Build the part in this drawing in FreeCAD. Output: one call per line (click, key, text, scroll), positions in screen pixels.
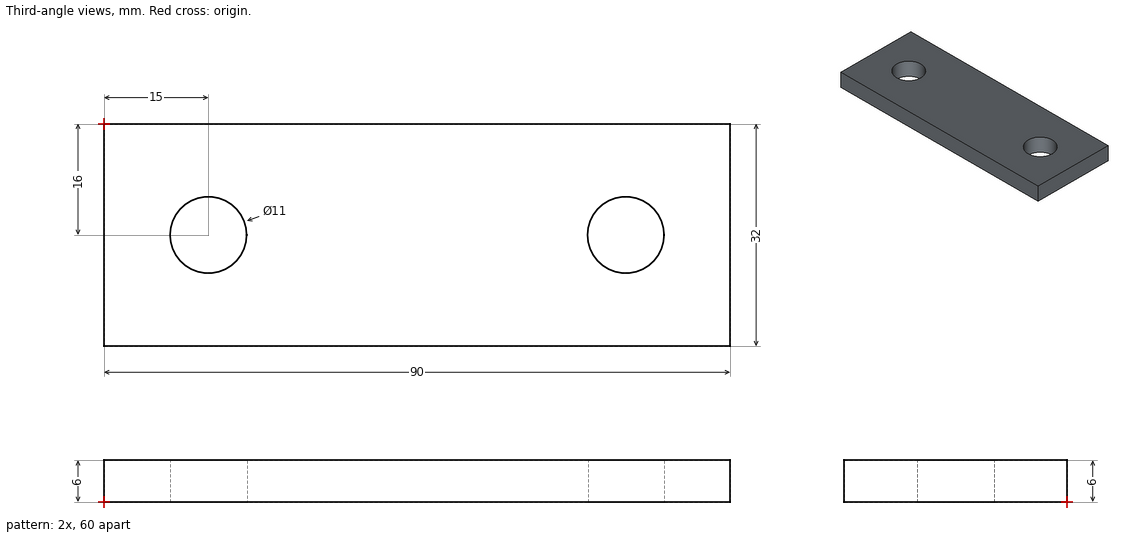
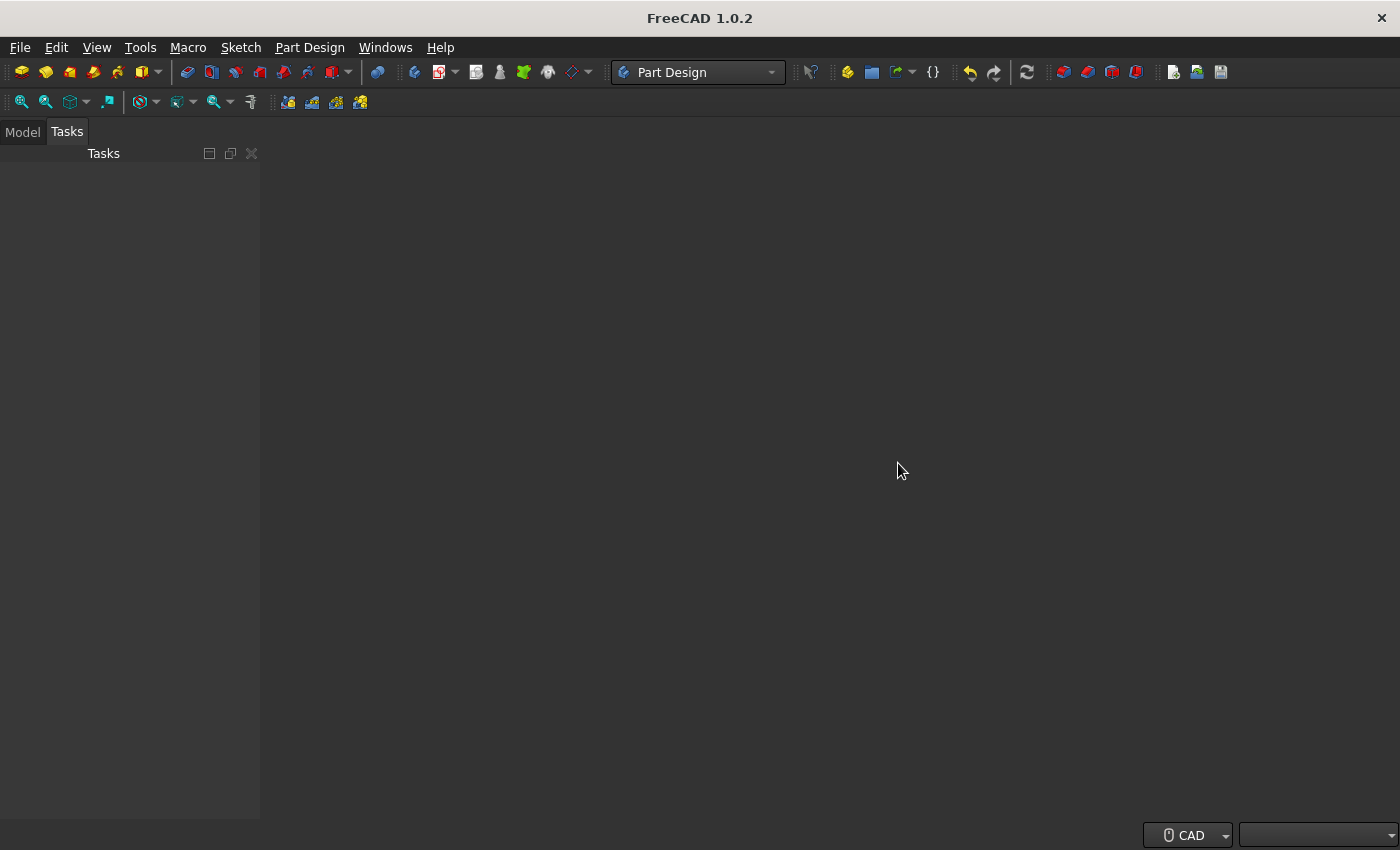
key(ctrl+n)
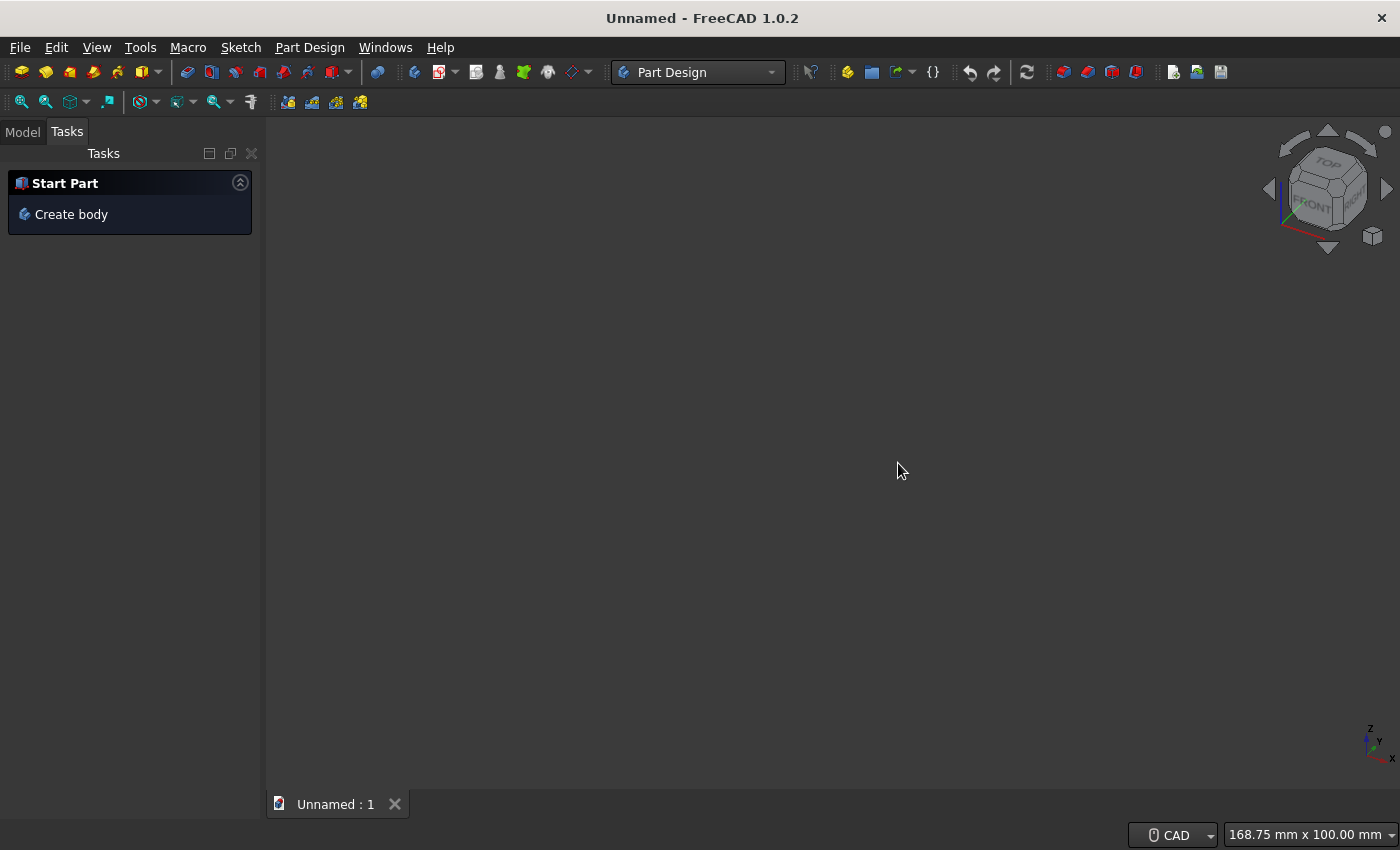
click(440, 72)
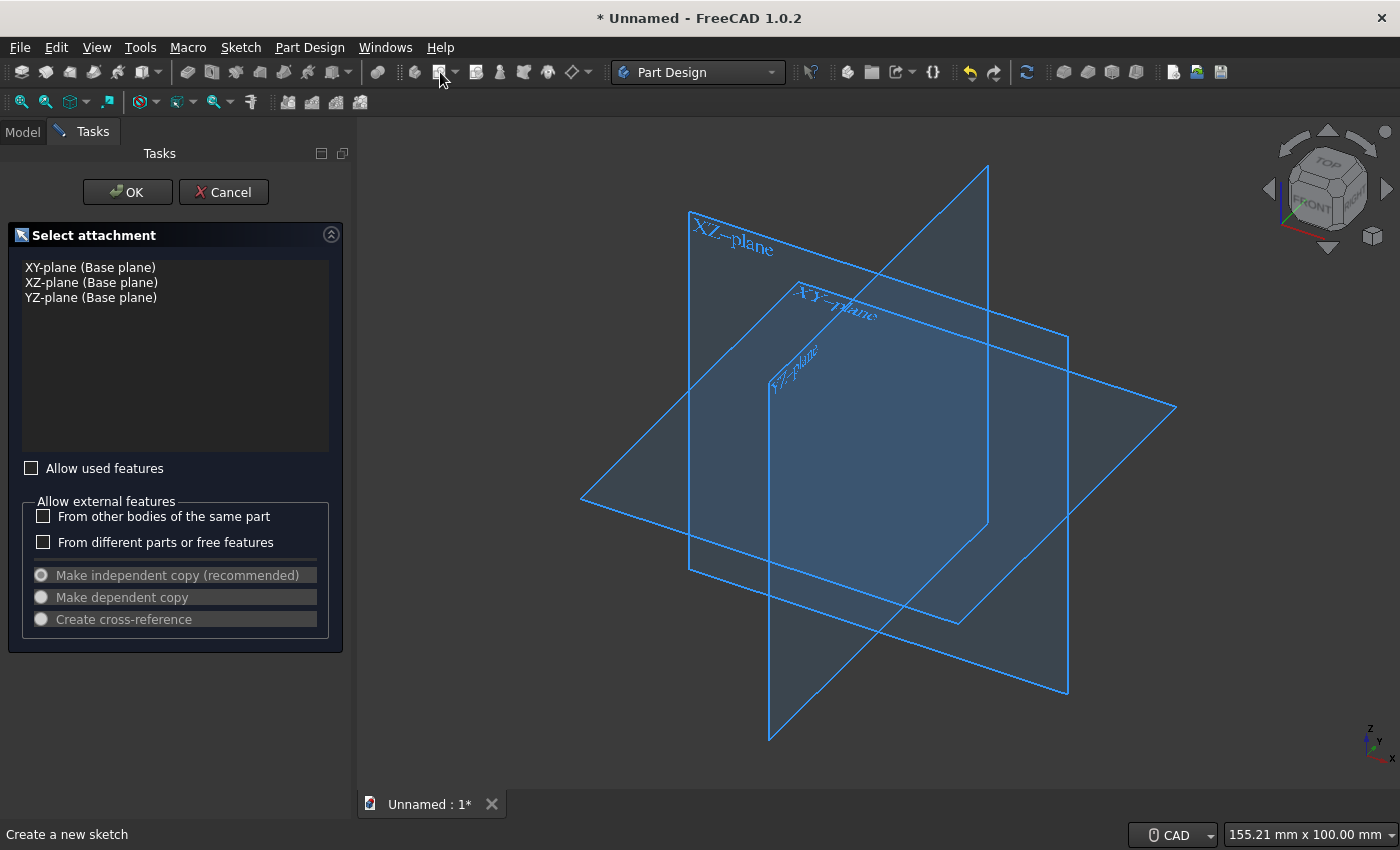
click(82, 268)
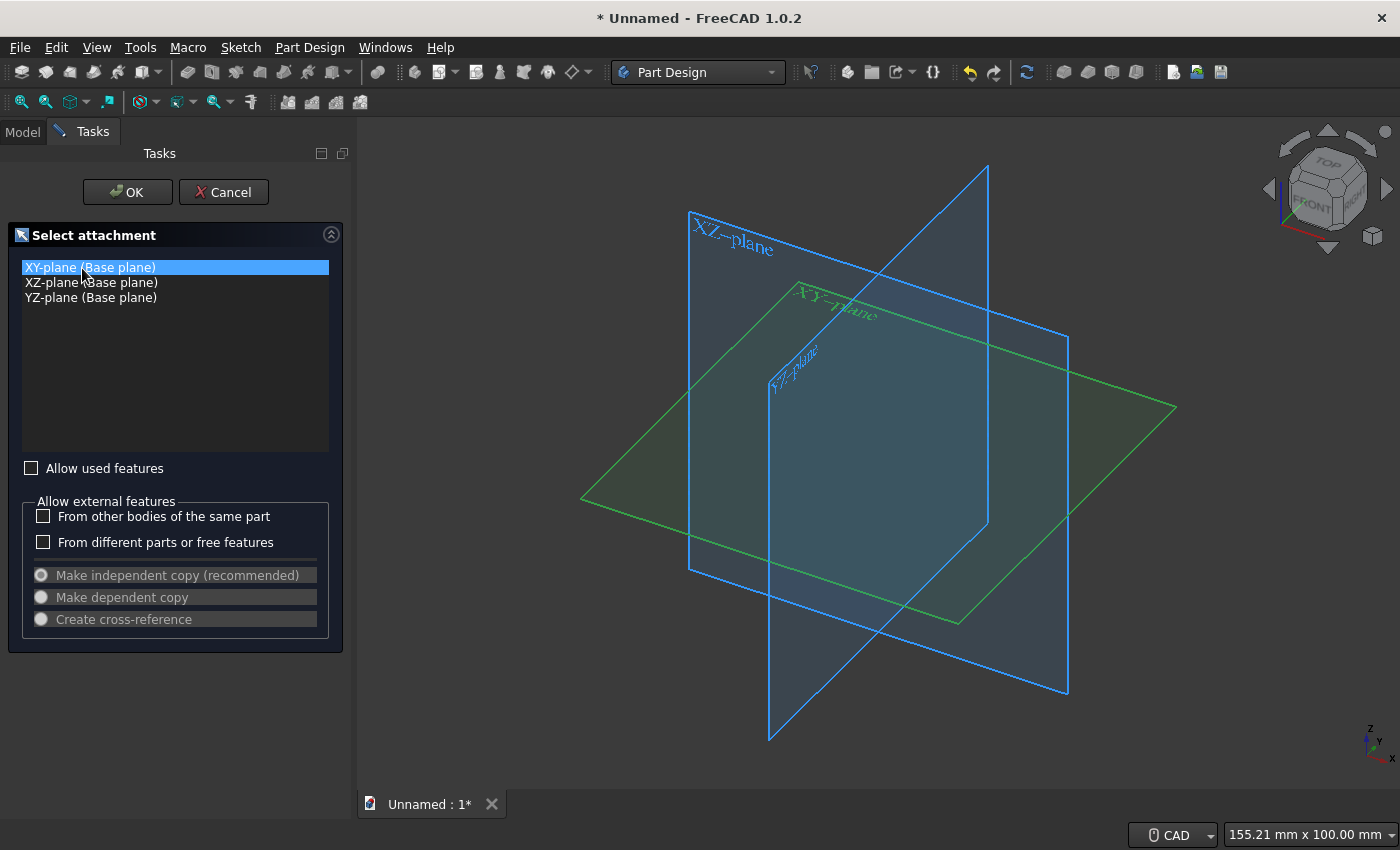
click(128, 192)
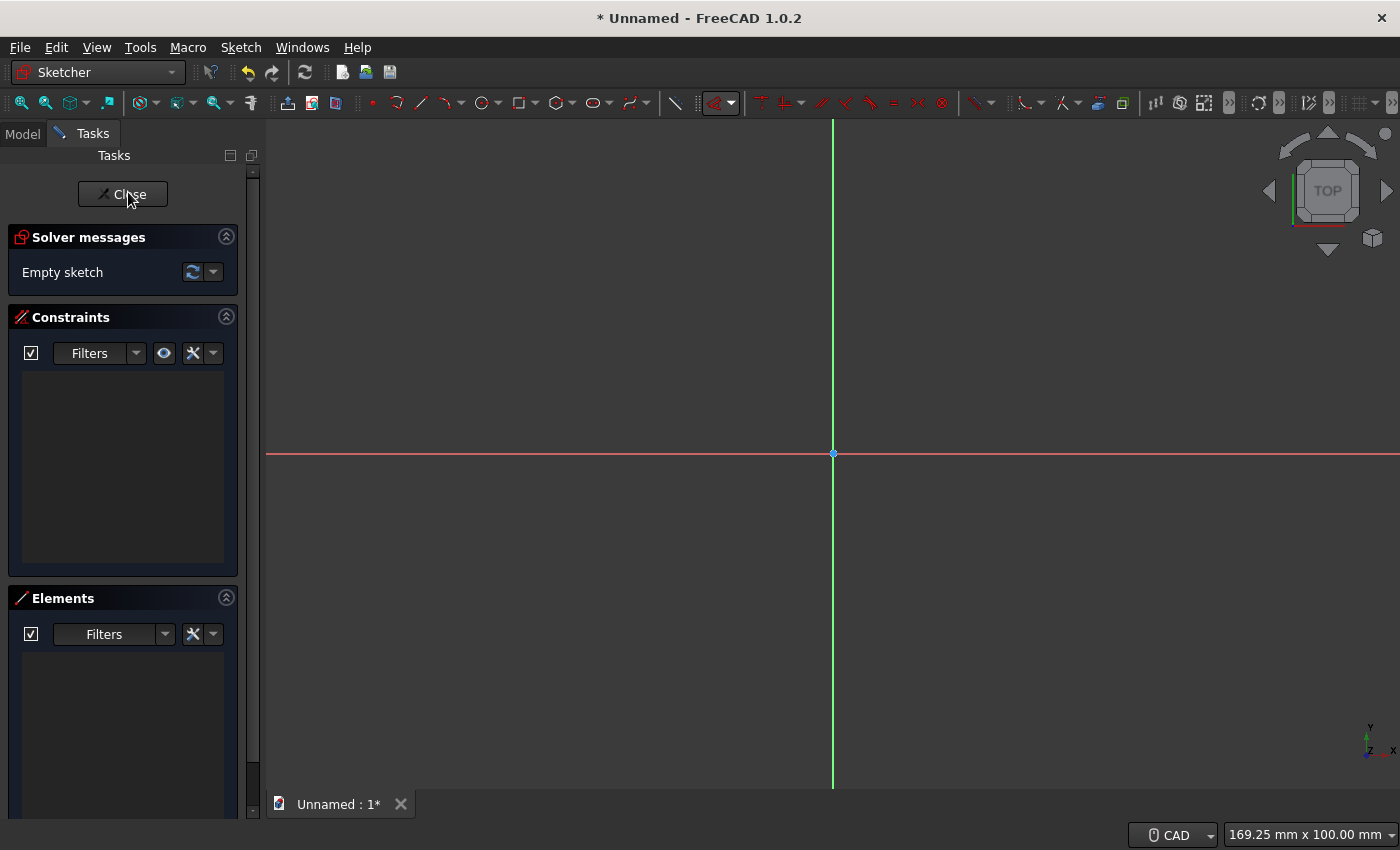
scroll(294, 236, down, 2)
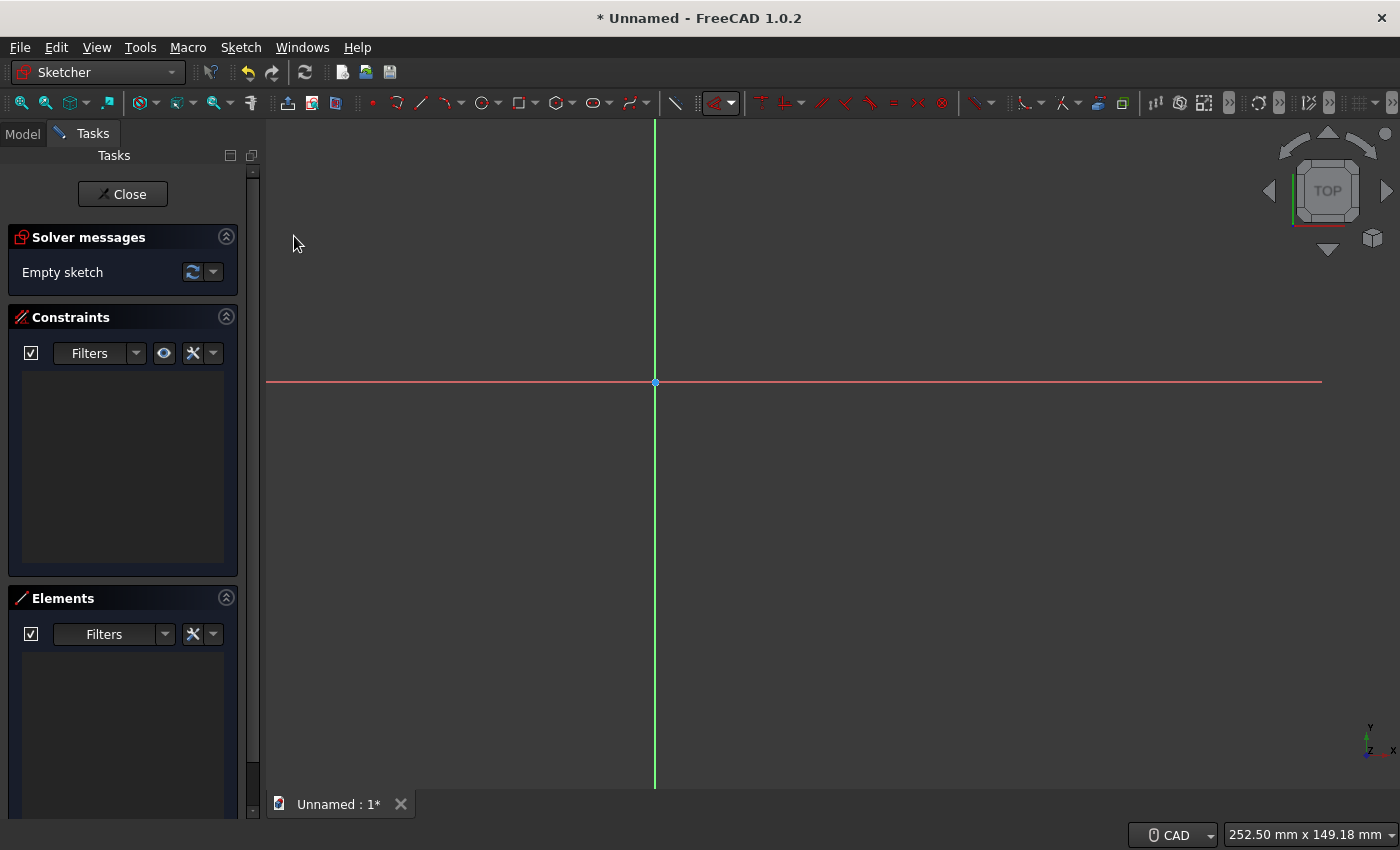
scroll(1046, 454, up, 2)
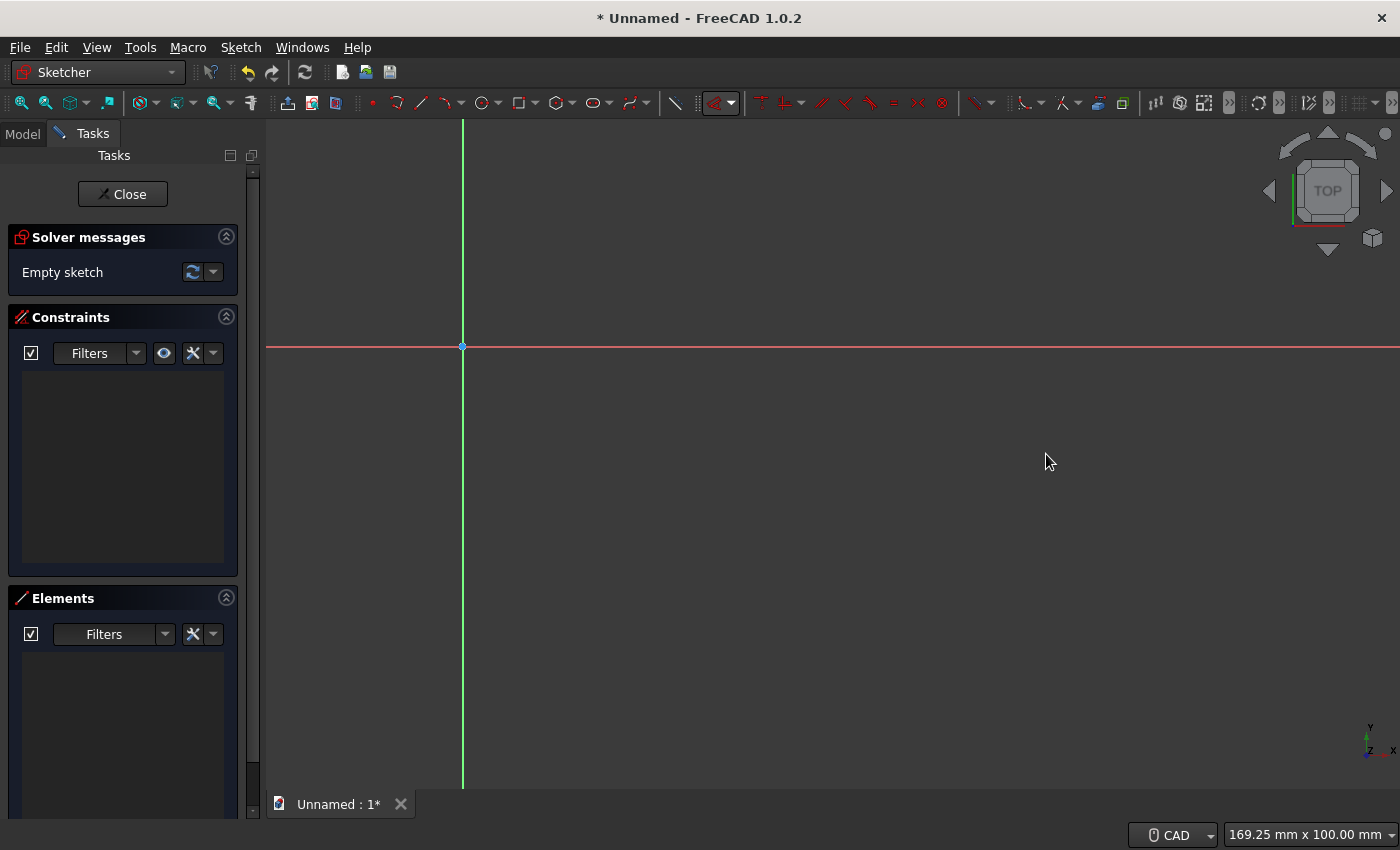
click(520, 104)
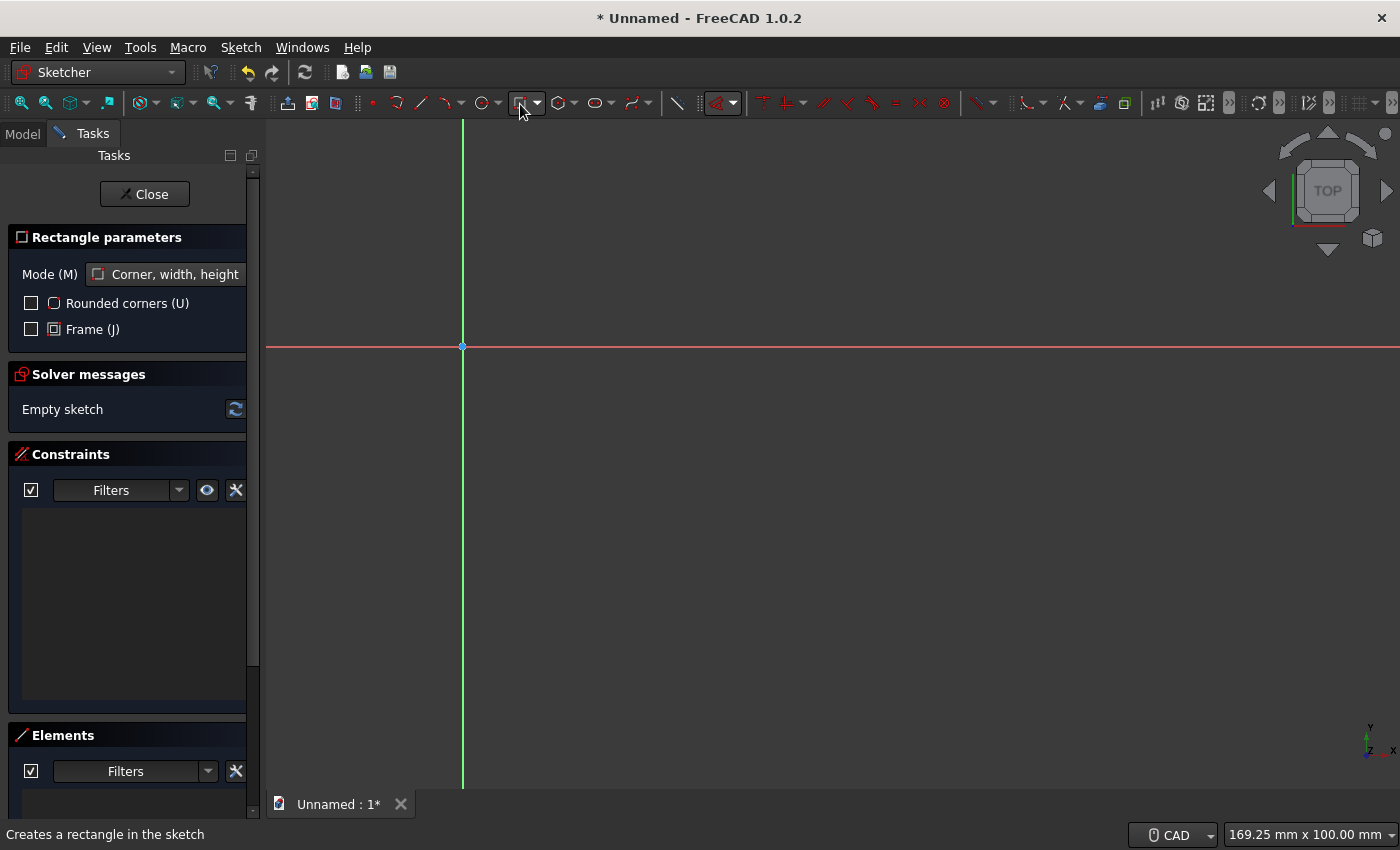
click(463, 347)
move(1066, 561)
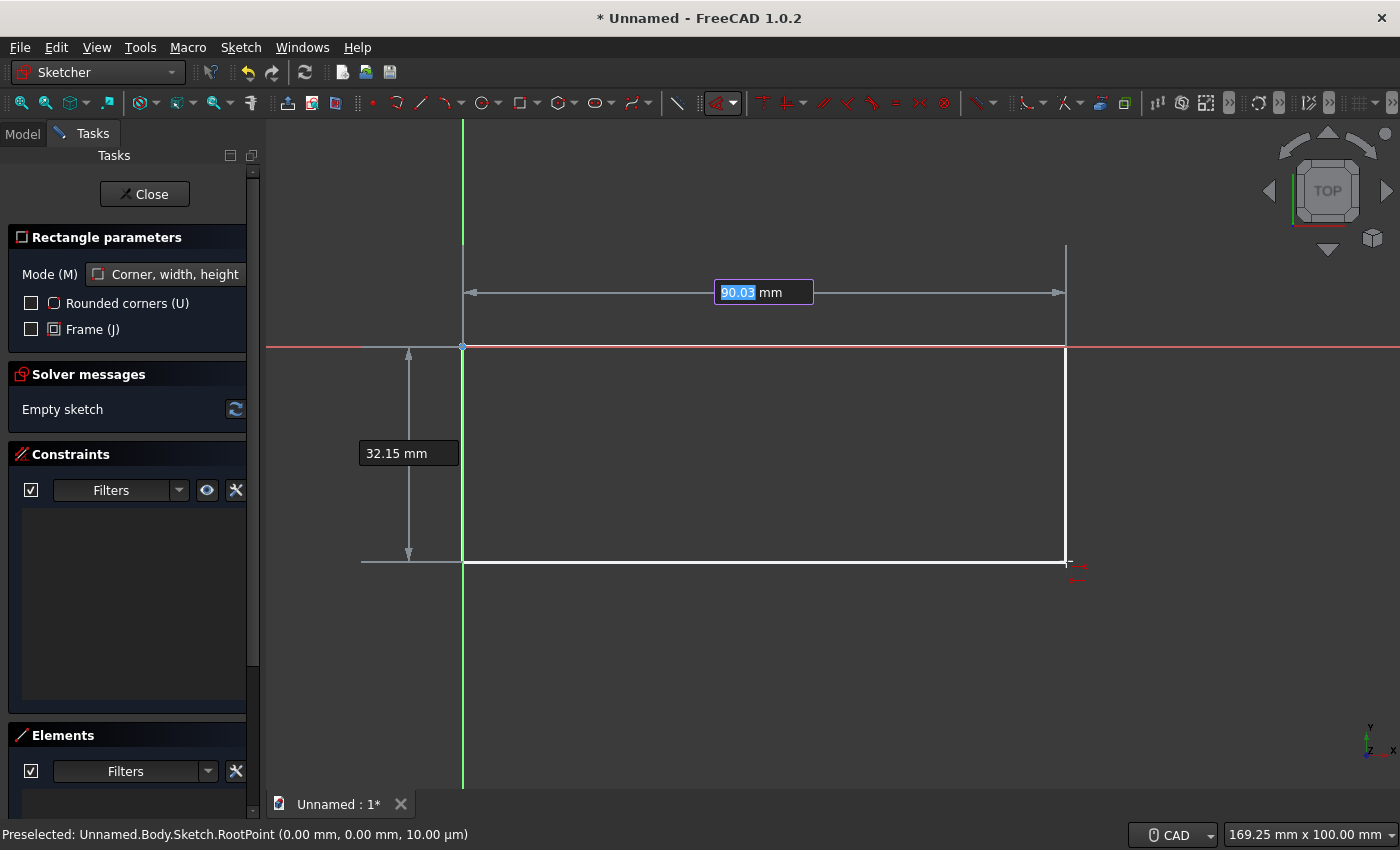
text(90)
key(Tab)
text(32)
key(Return)
key(Escape)